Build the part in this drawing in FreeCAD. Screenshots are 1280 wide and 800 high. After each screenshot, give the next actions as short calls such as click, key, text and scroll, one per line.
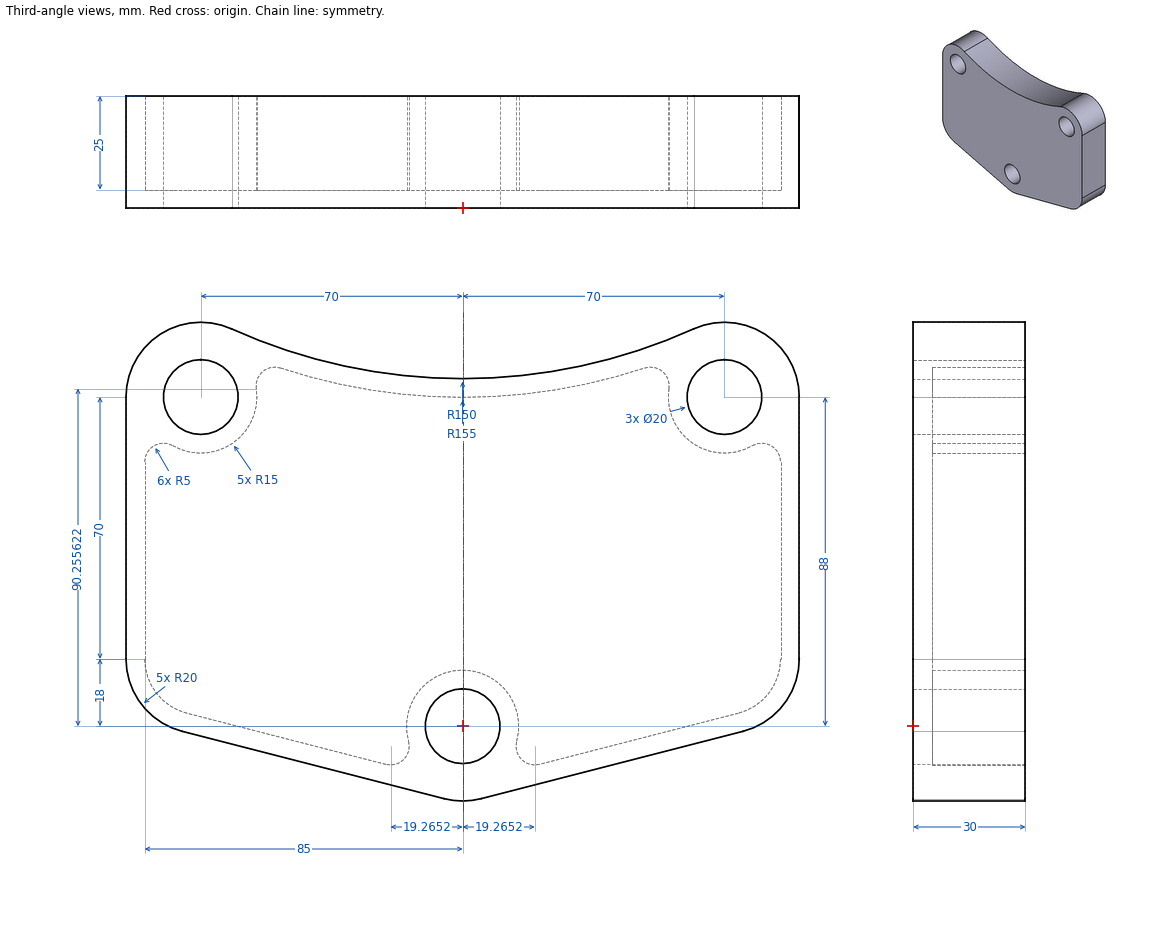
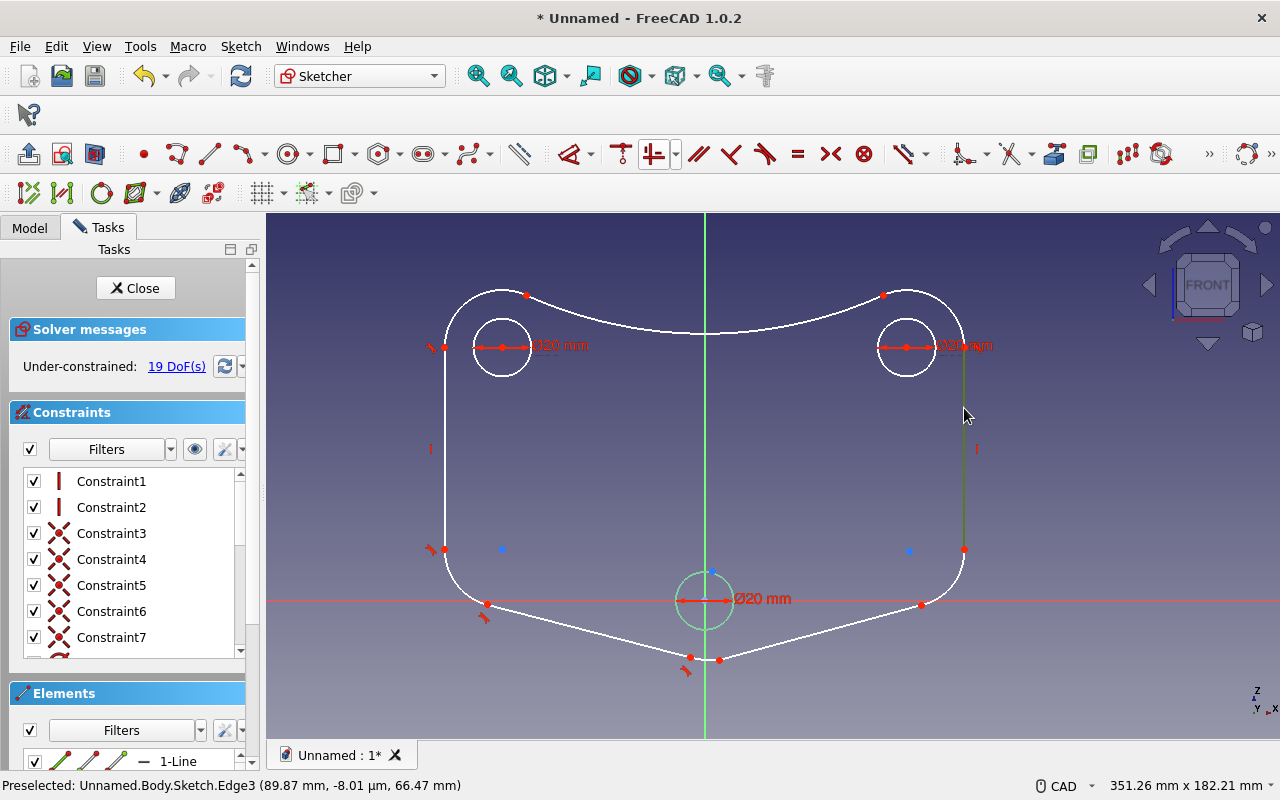
click(960, 572)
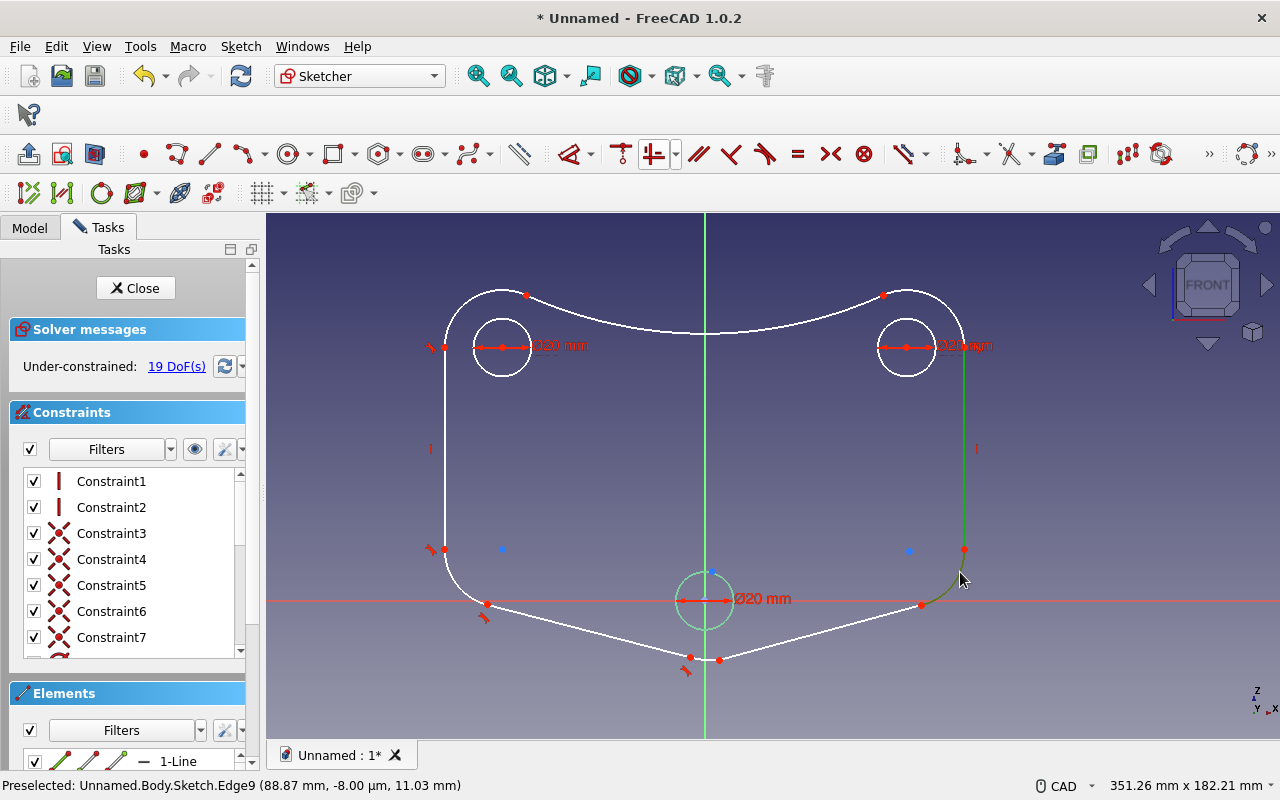
click(765, 154)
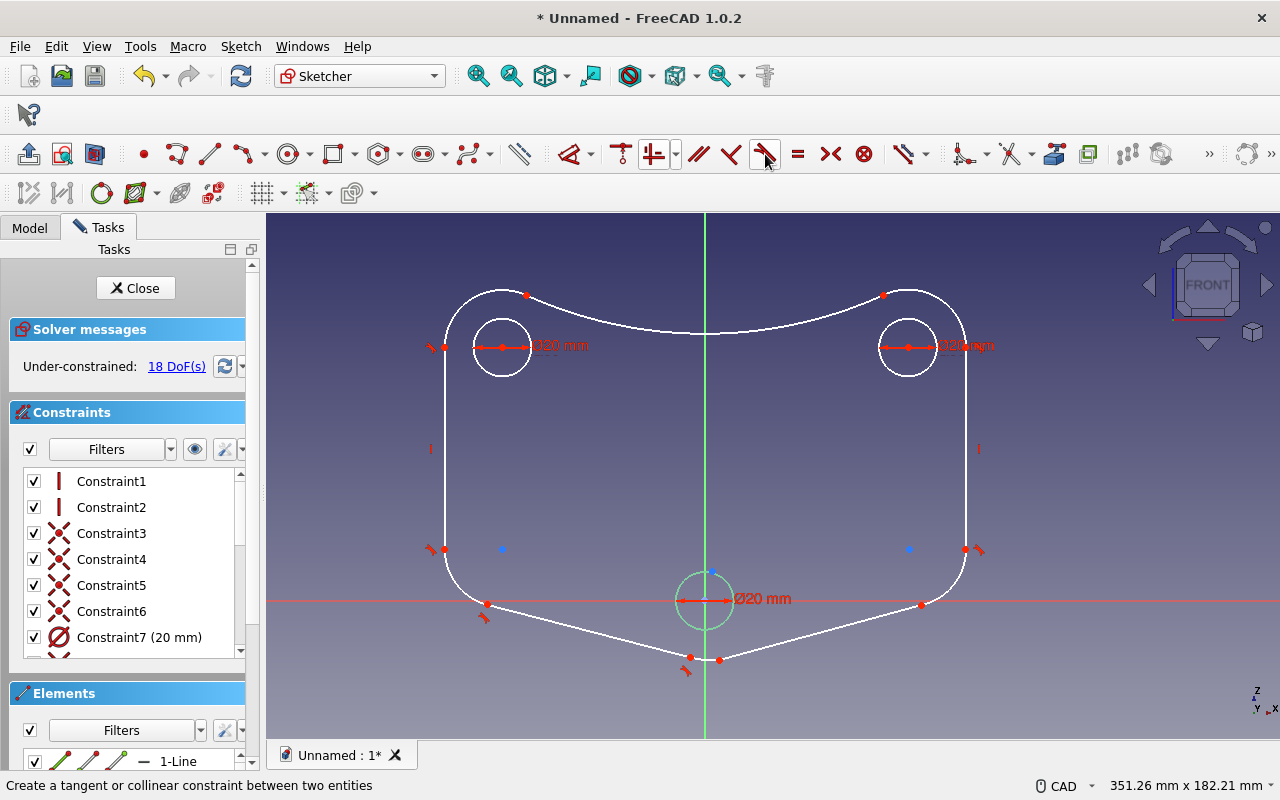
click(861, 622)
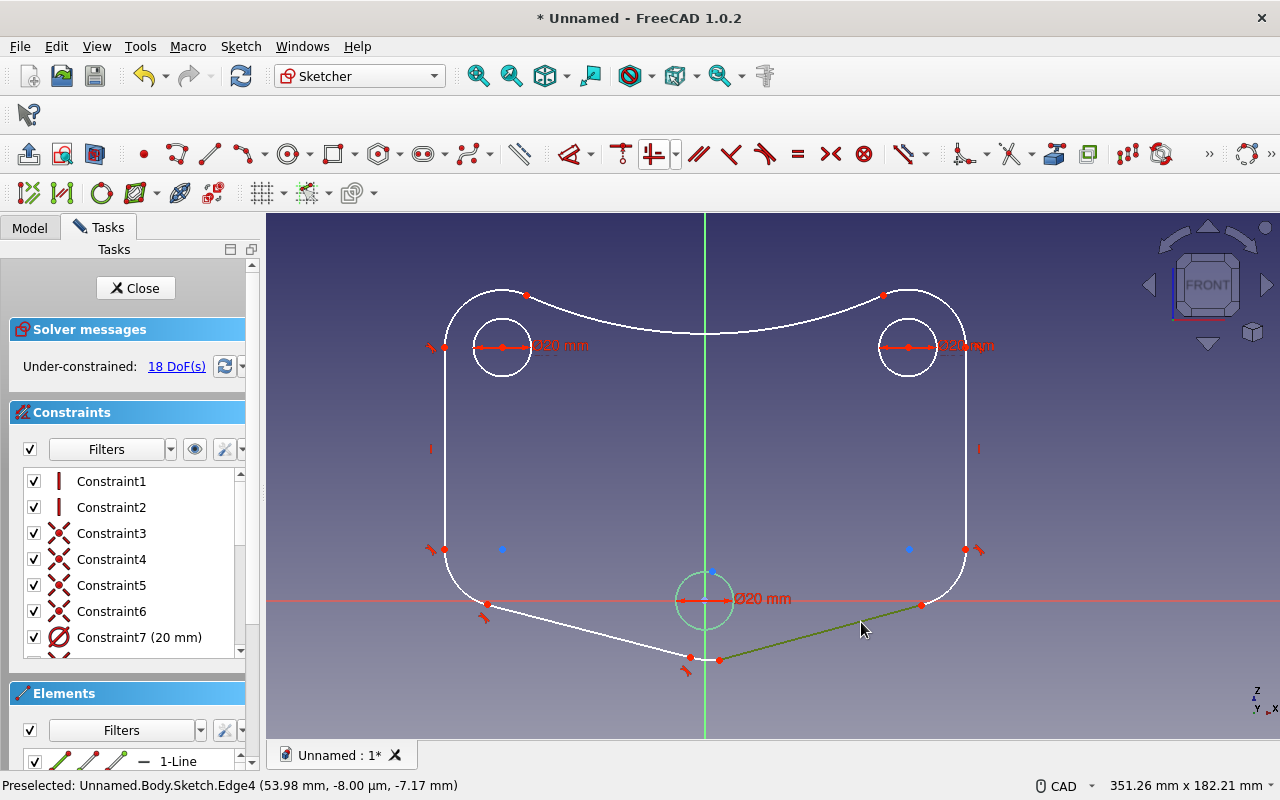
click(961, 572)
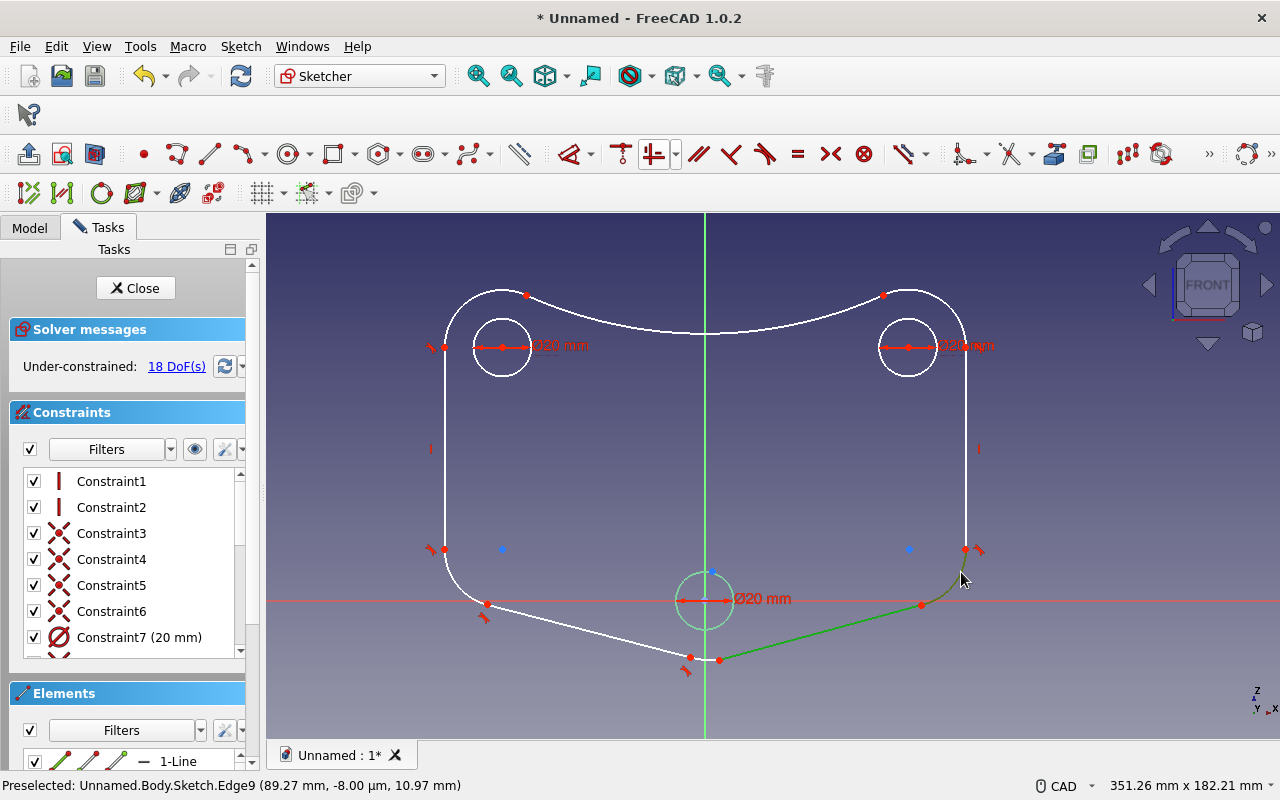
click(765, 154)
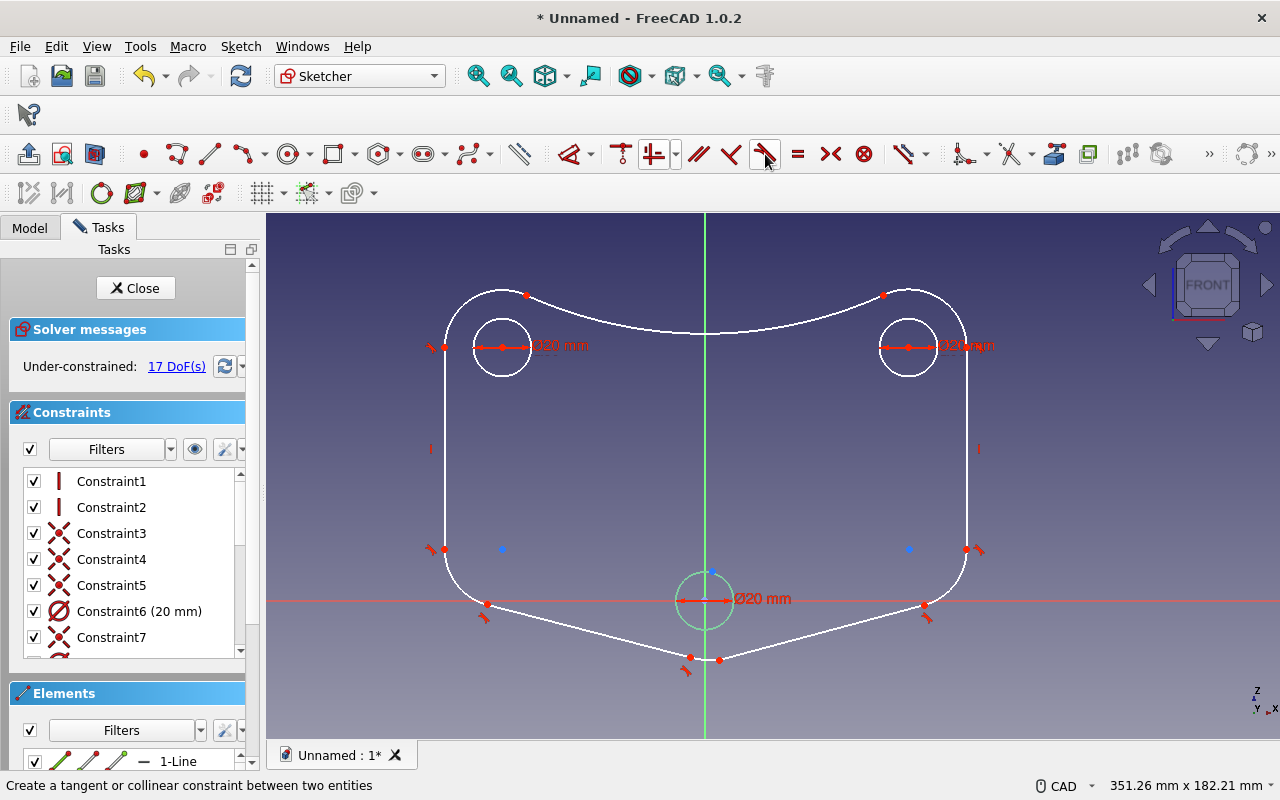
click(863, 622)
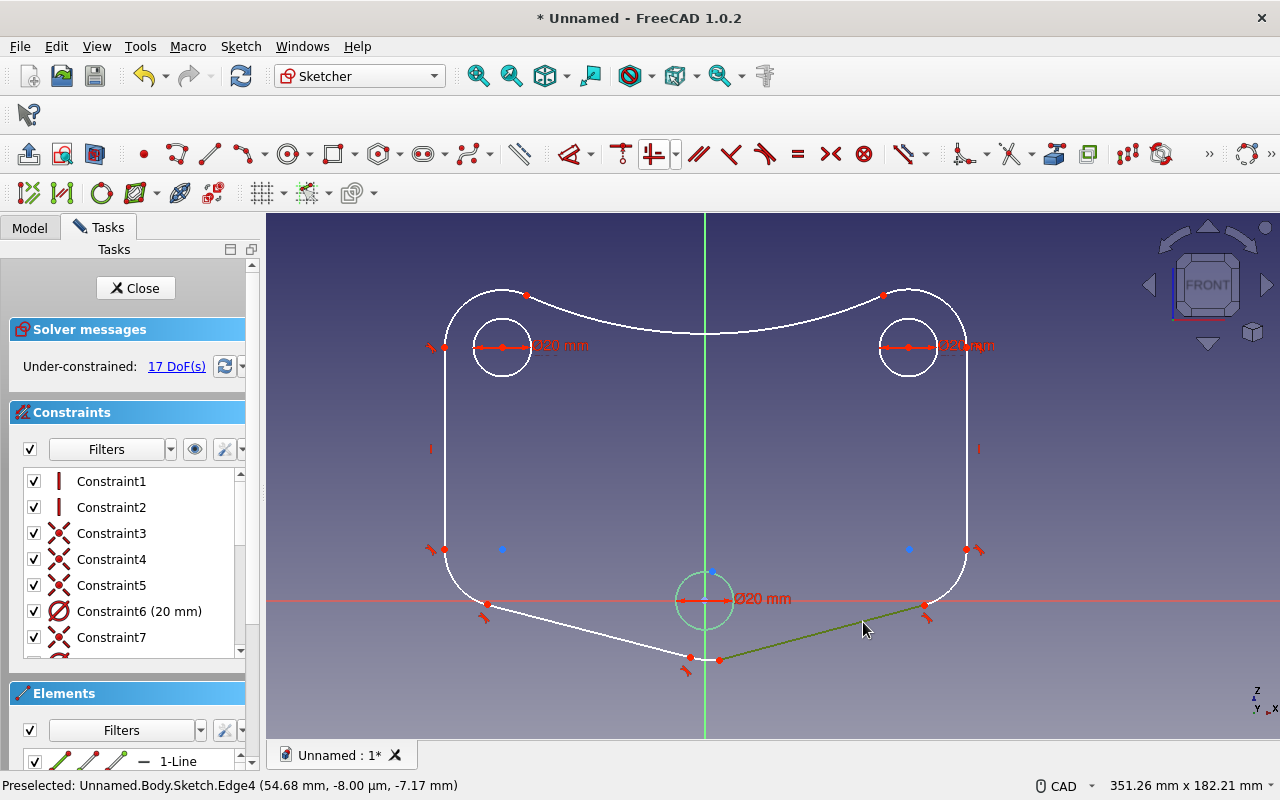
click(705, 660)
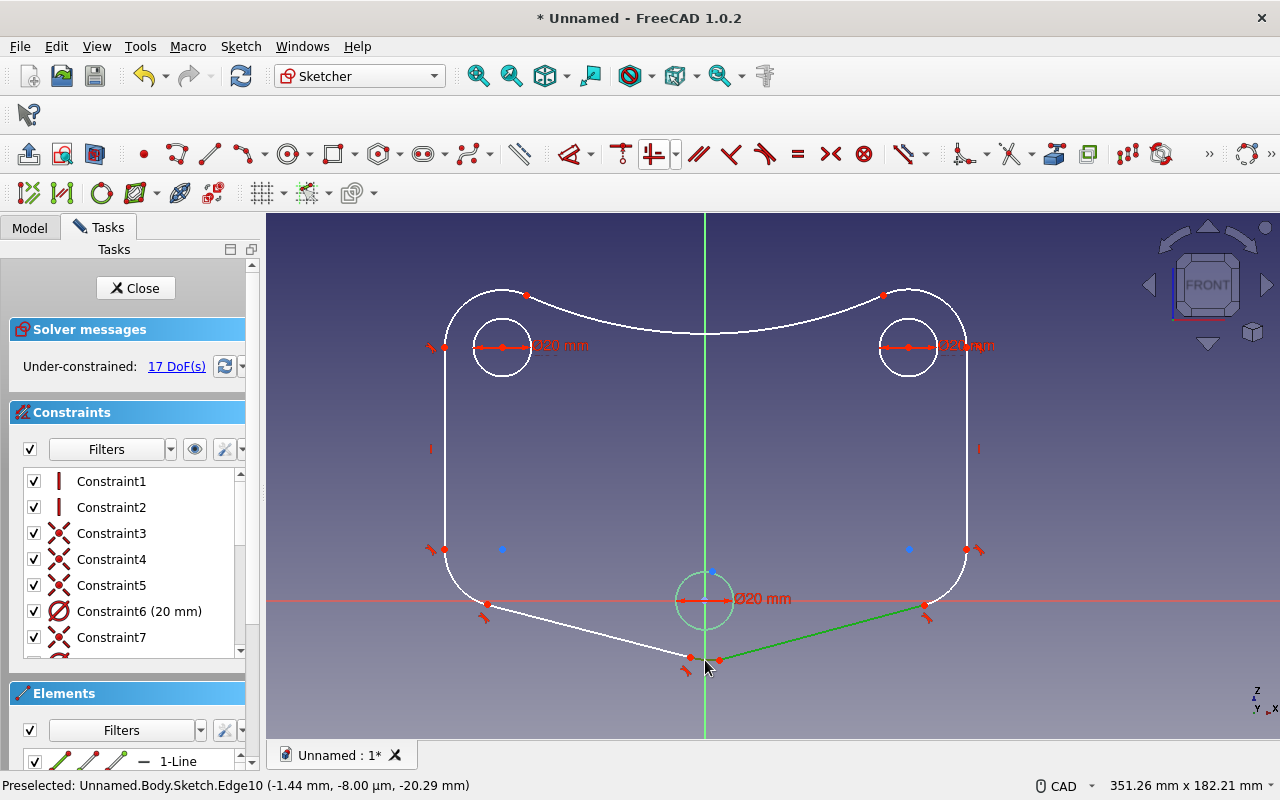
click(765, 154)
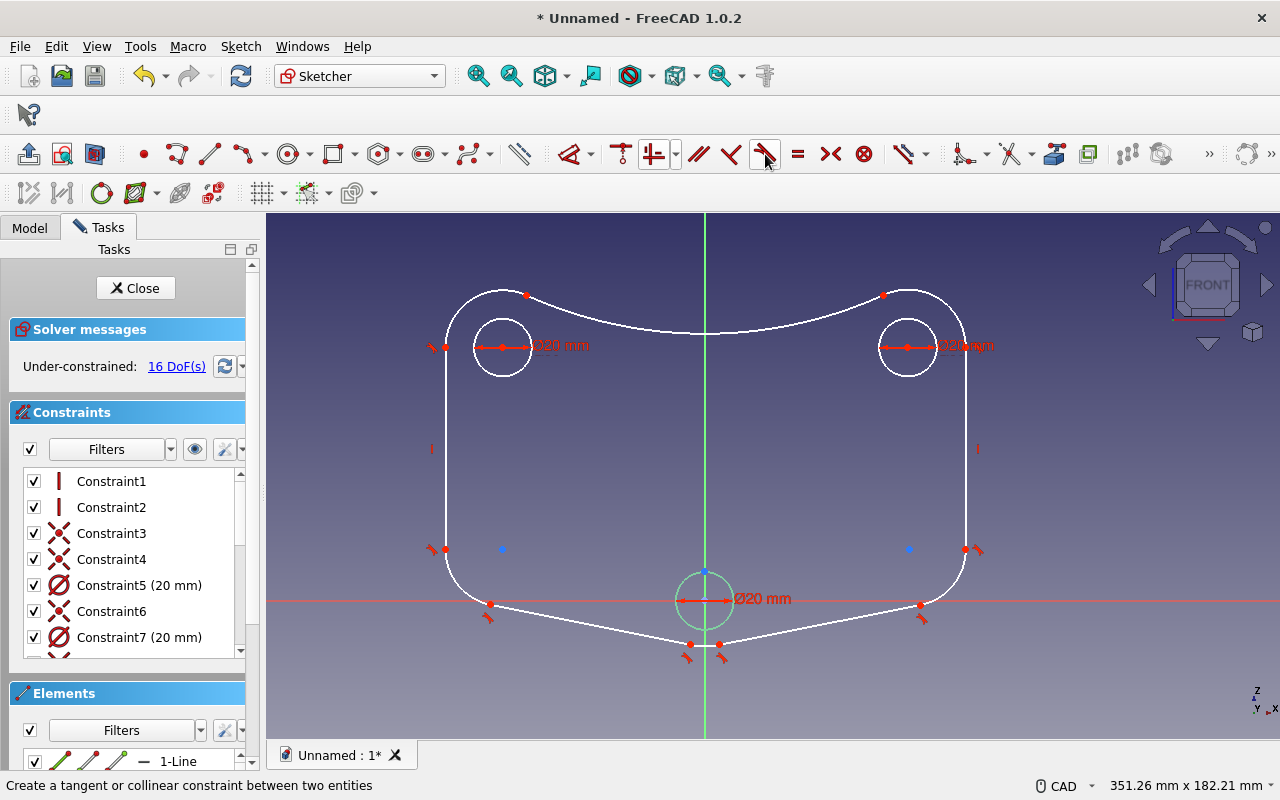
click(493, 291)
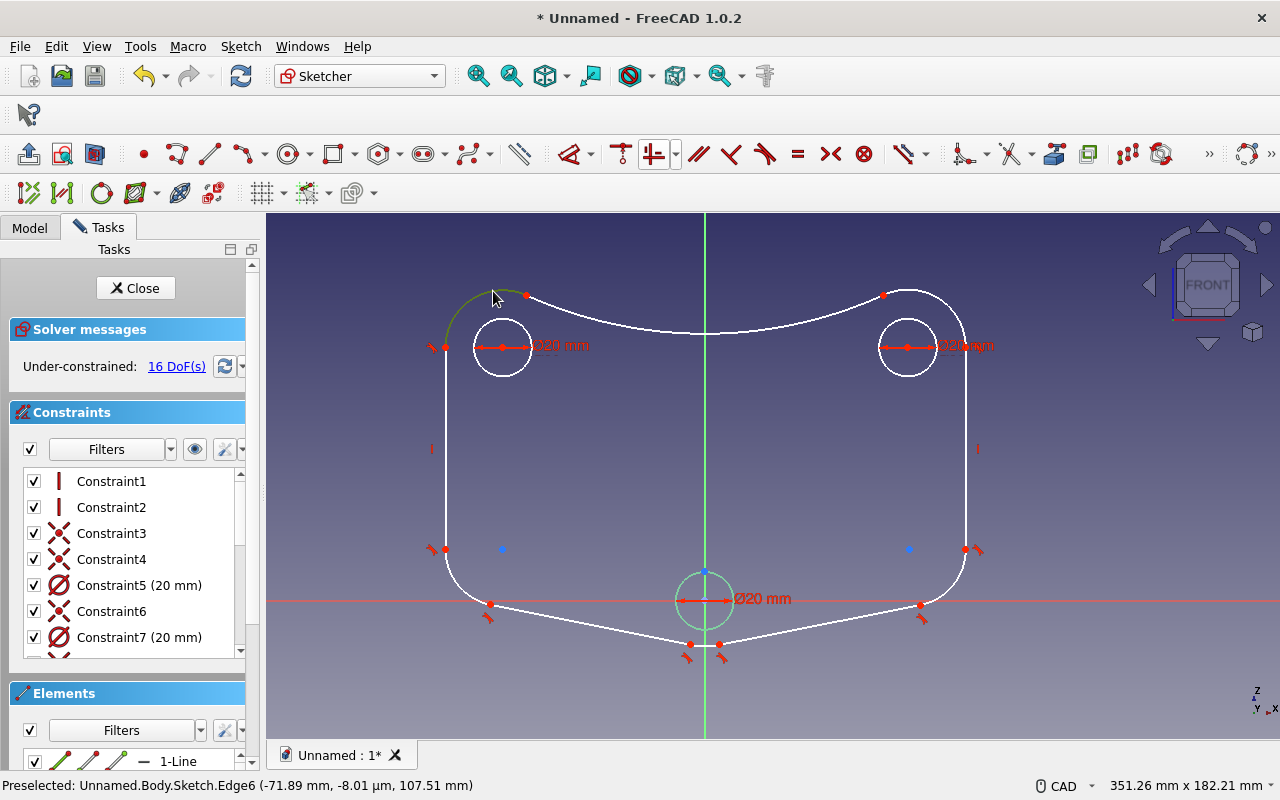
click(631, 328)